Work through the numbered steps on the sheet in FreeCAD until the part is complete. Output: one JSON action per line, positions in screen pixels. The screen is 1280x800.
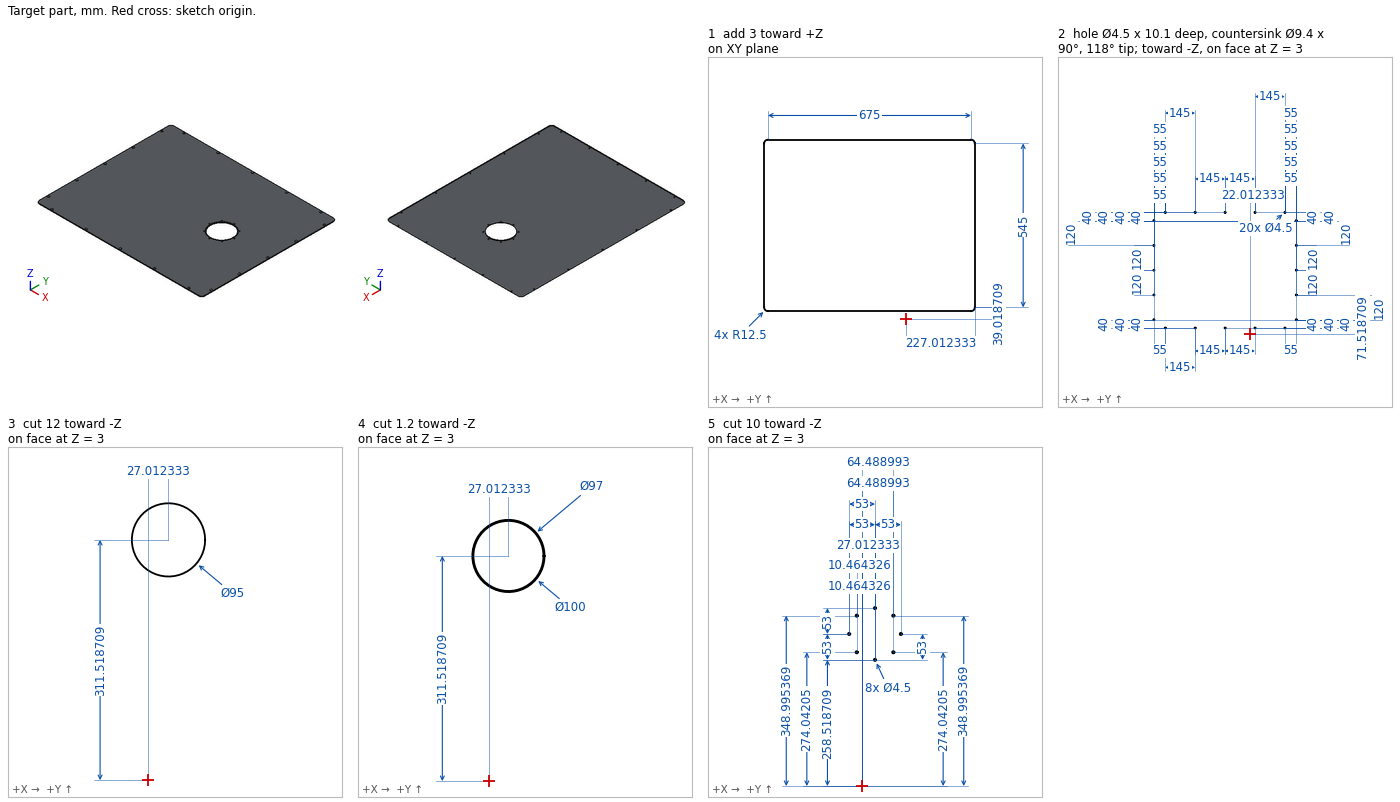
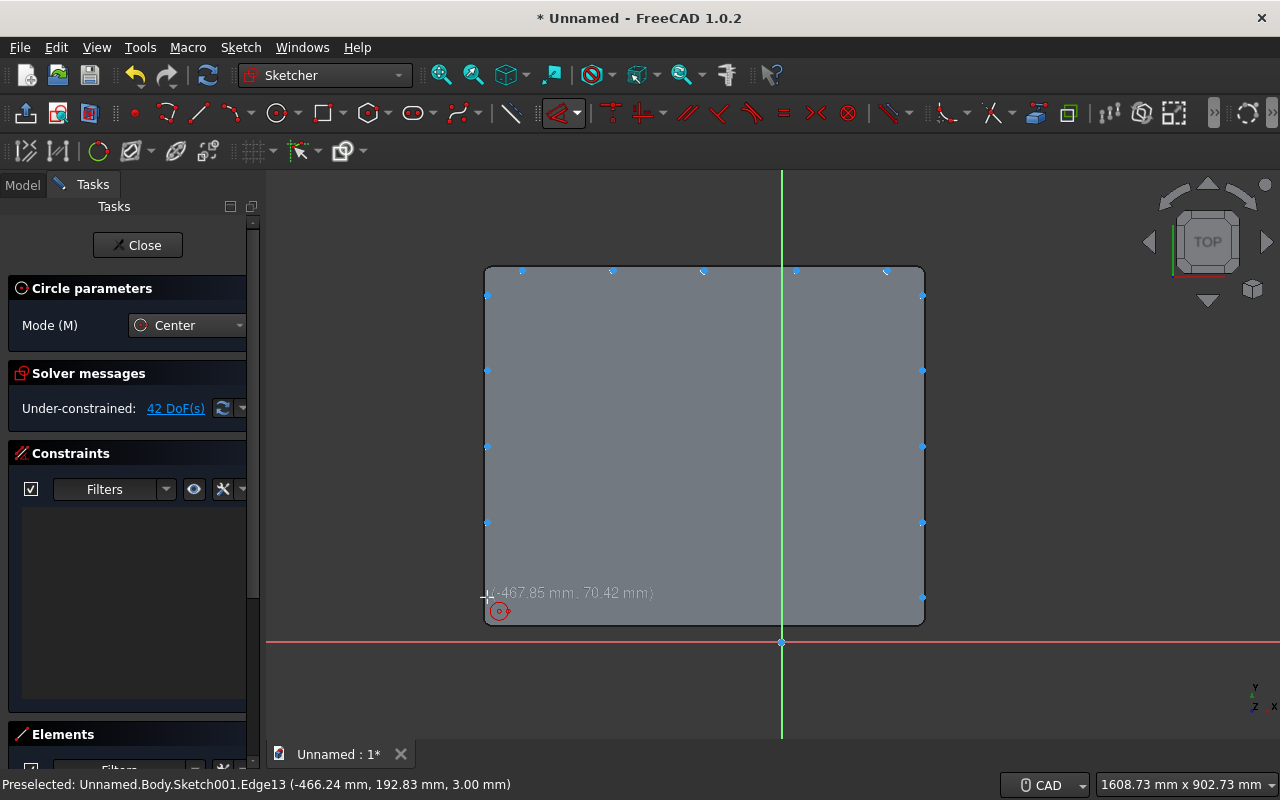
{"action": "left_click", "coordinate": [487, 597]}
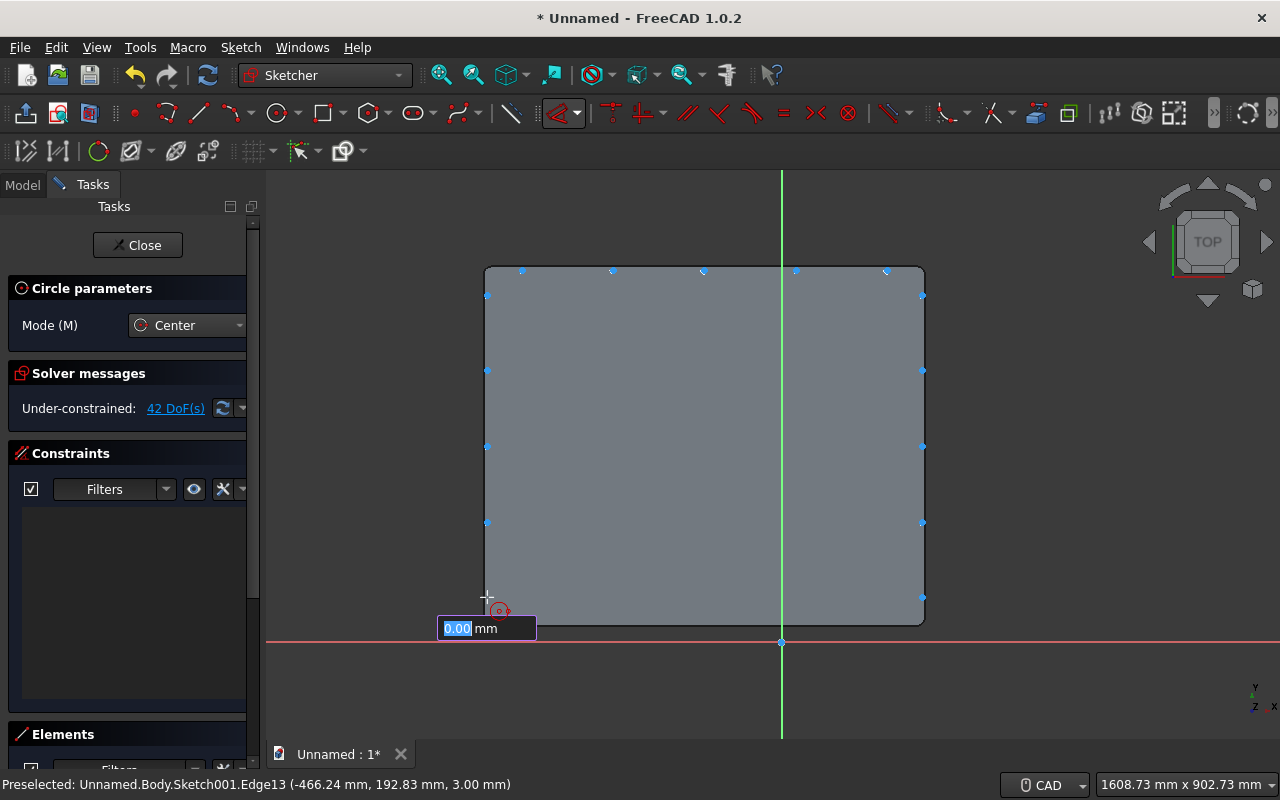
{"action": "scroll", "coordinate": [488, 596], "scroll_direction": "up", "scroll_amount": 13}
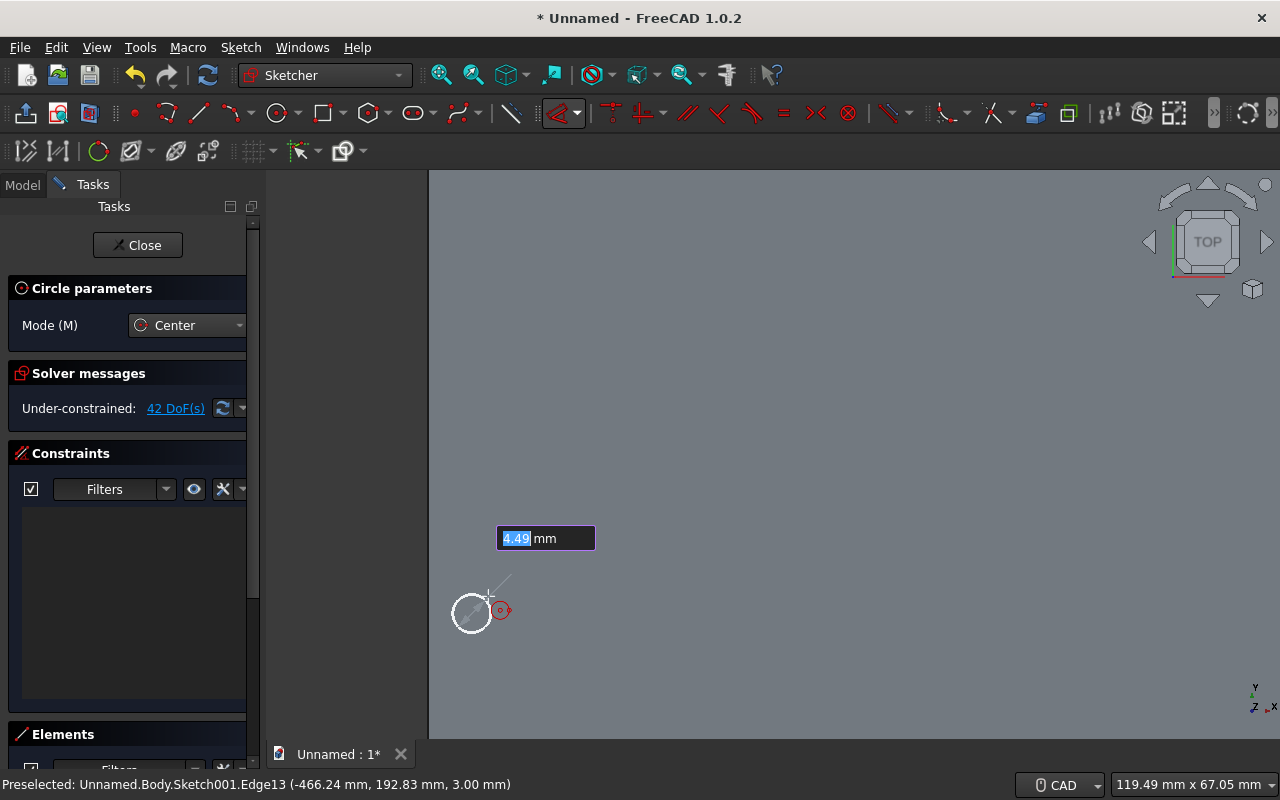
{"action": "left_click", "coordinate": [484, 591]}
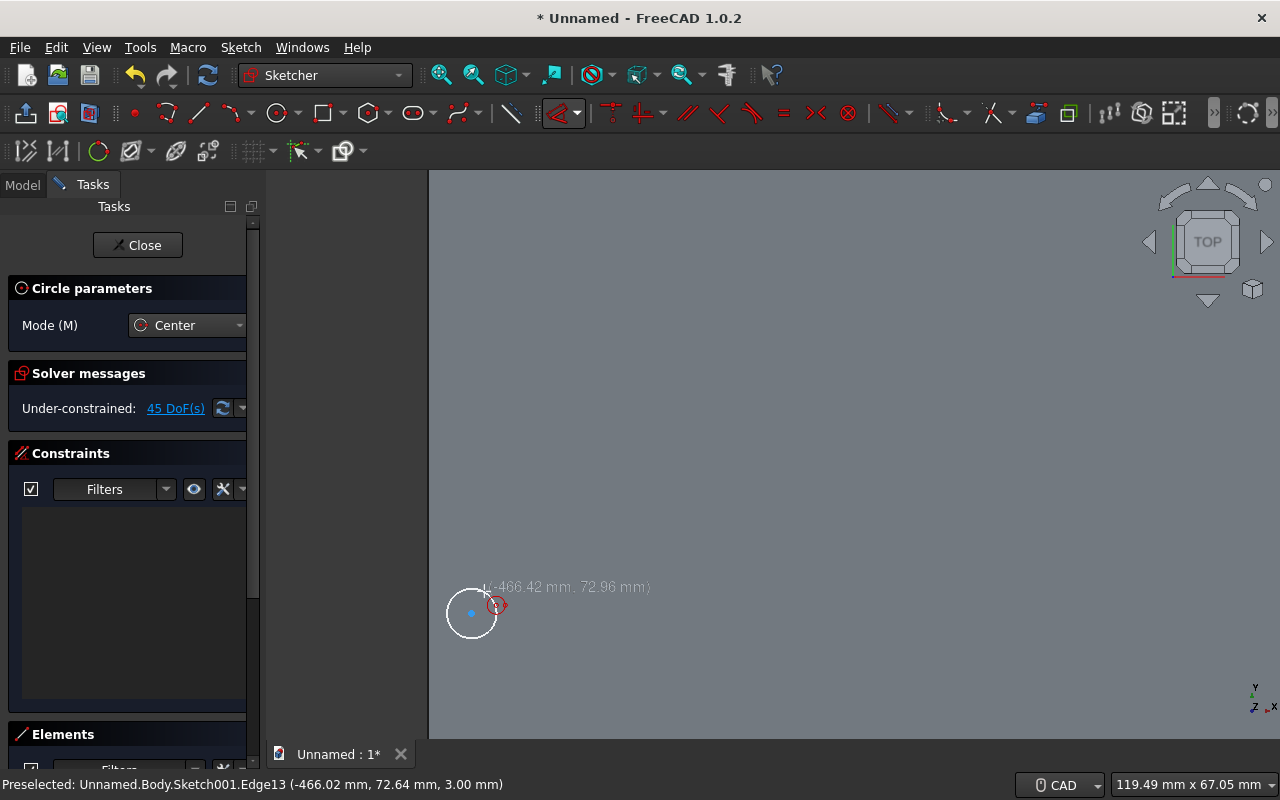
{"action": "scroll", "coordinate": [488, 596], "scroll_direction": "down", "scroll_amount": 13}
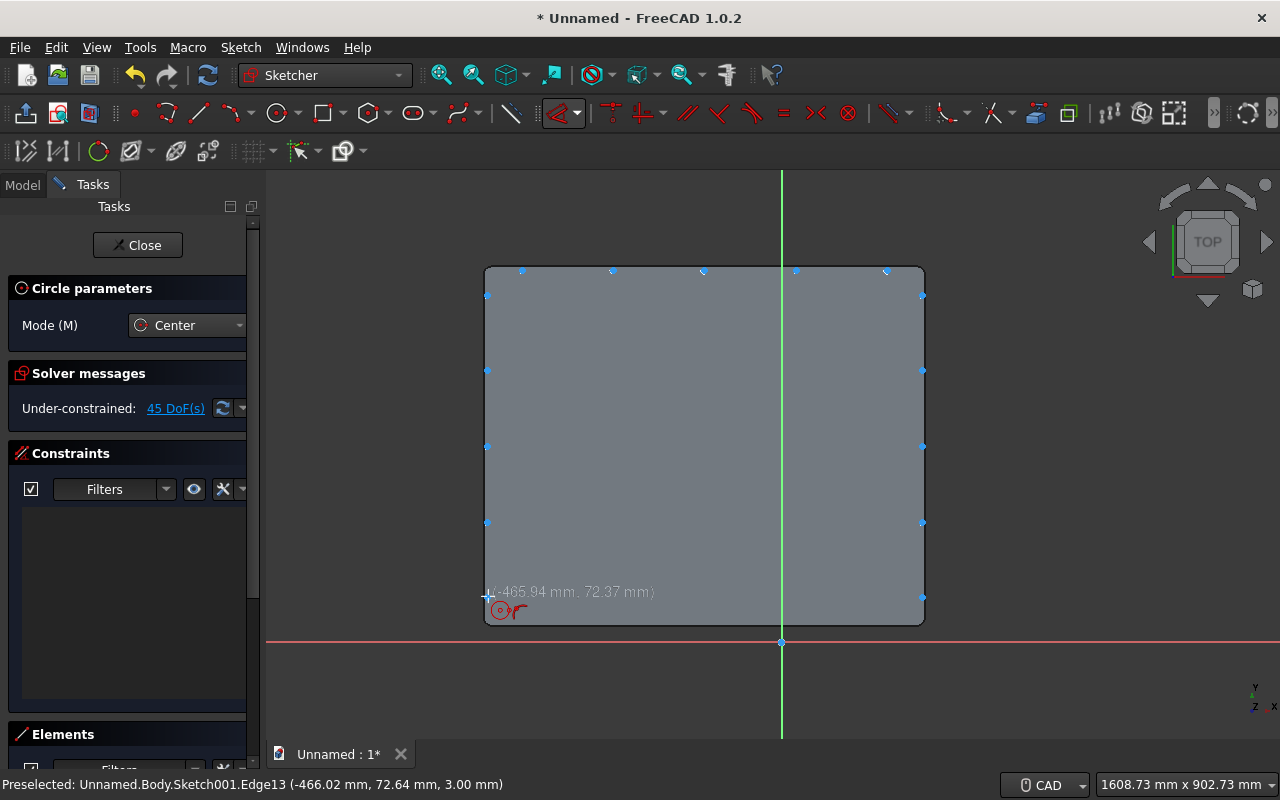
{"action": "scroll", "coordinate": [522, 623], "scroll_direction": "up", "scroll_amount": 14}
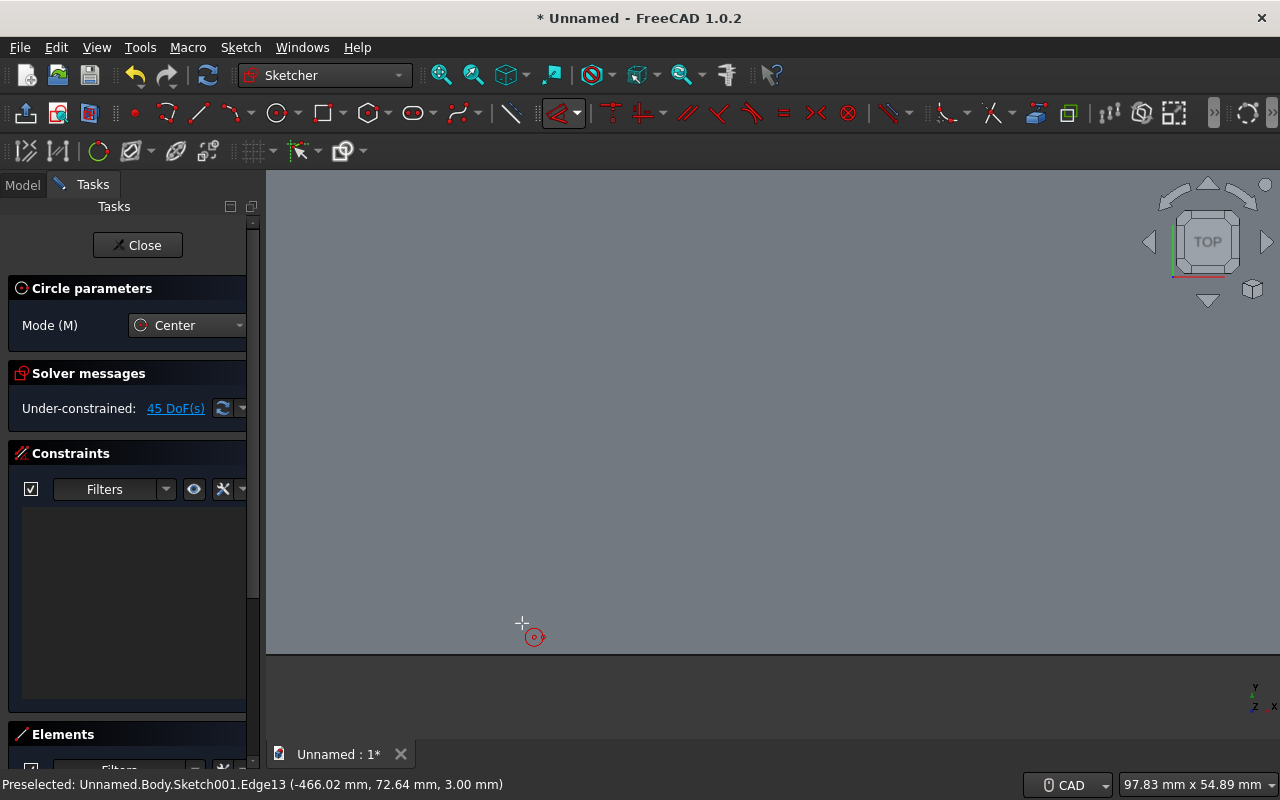
{"action": "scroll", "coordinate": [522, 623], "scroll_direction": "down", "scroll_amount": 14}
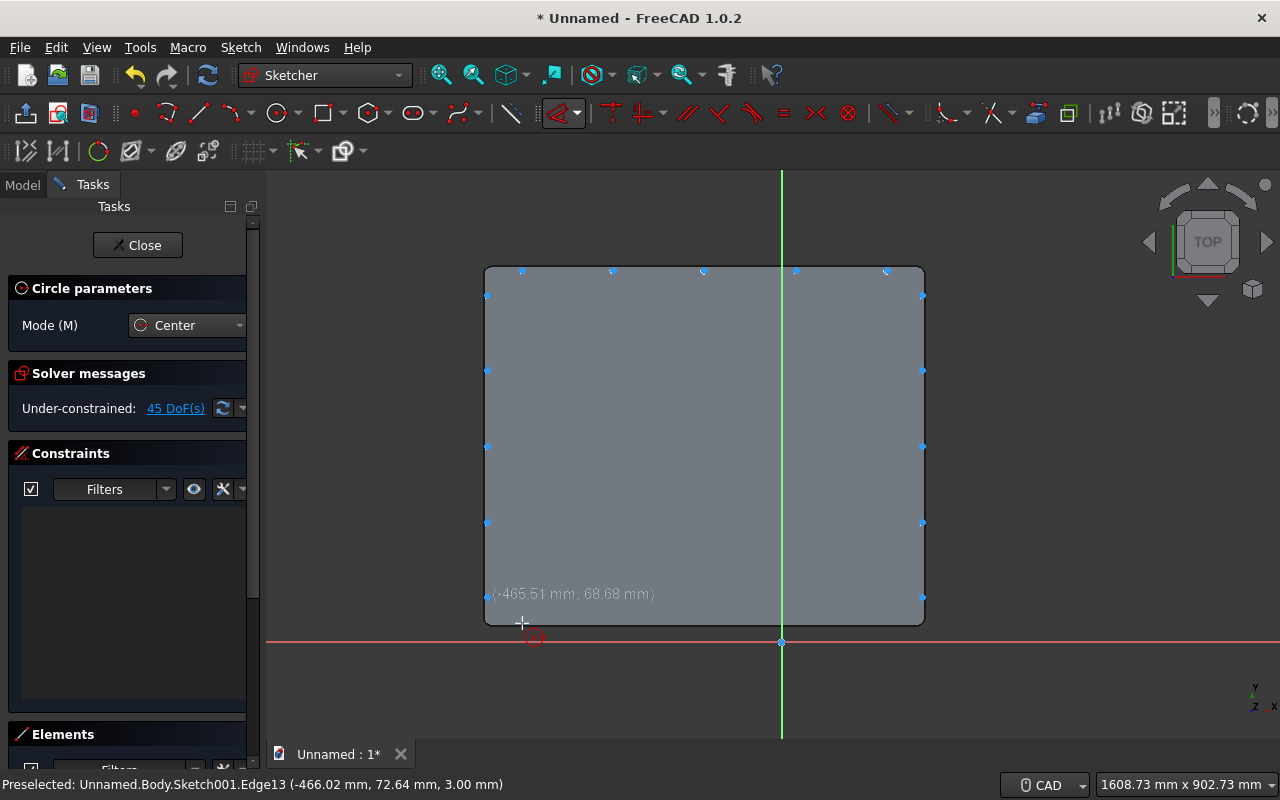
{"action": "left_click", "coordinate": [522, 623]}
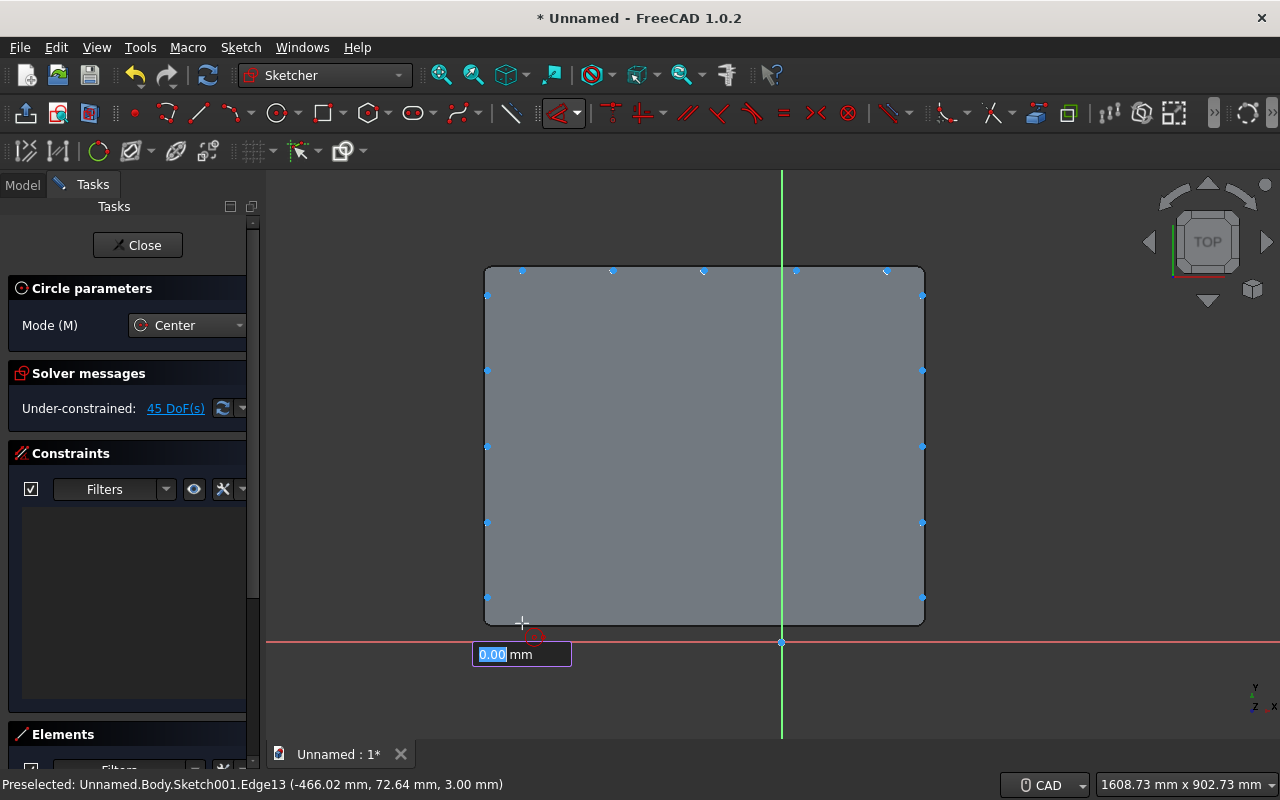
{"action": "scroll", "coordinate": [523, 622], "scroll_direction": "up", "scroll_amount": 13}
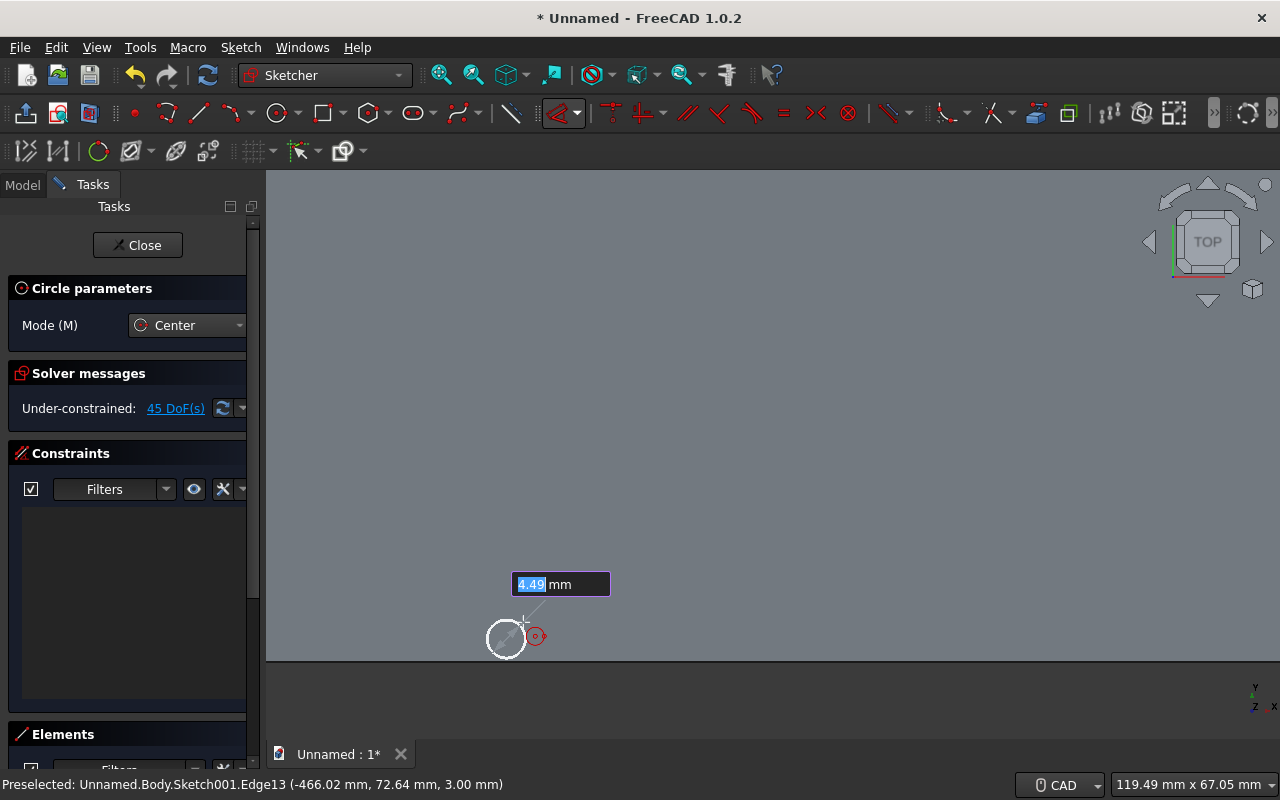
{"action": "left_click", "coordinate": [514, 606]}